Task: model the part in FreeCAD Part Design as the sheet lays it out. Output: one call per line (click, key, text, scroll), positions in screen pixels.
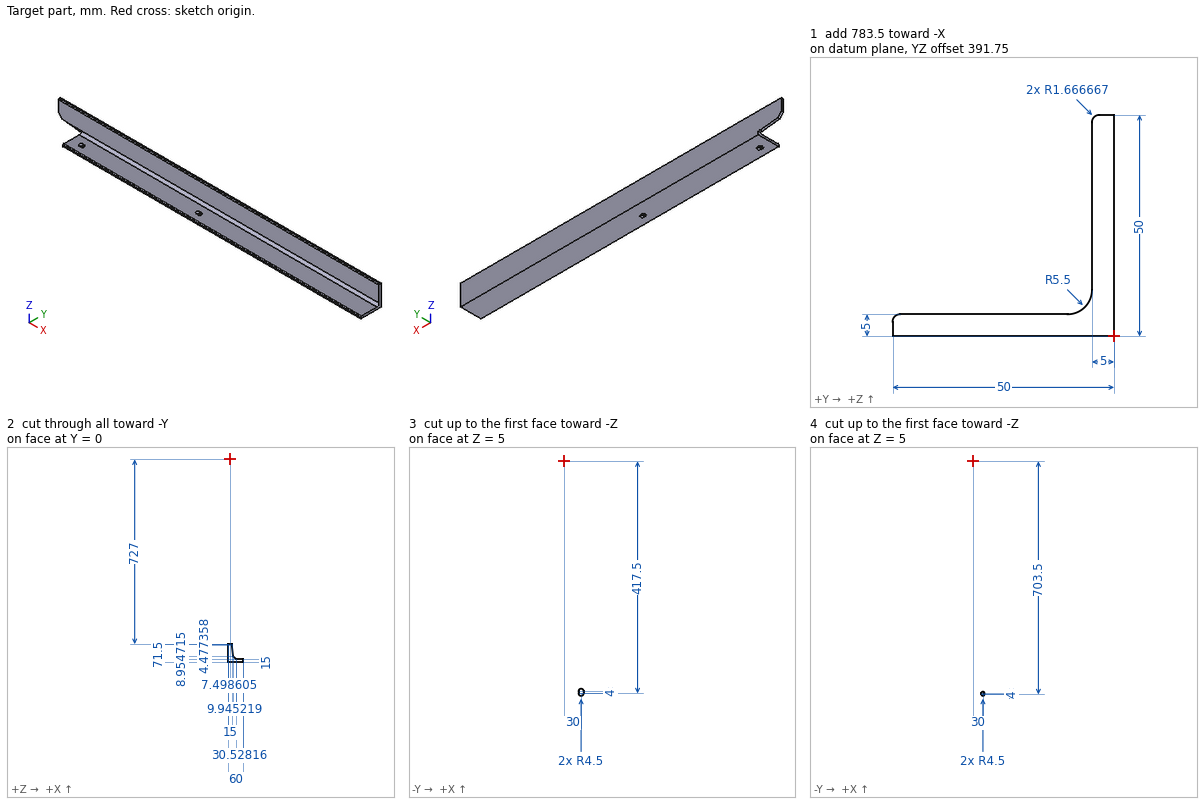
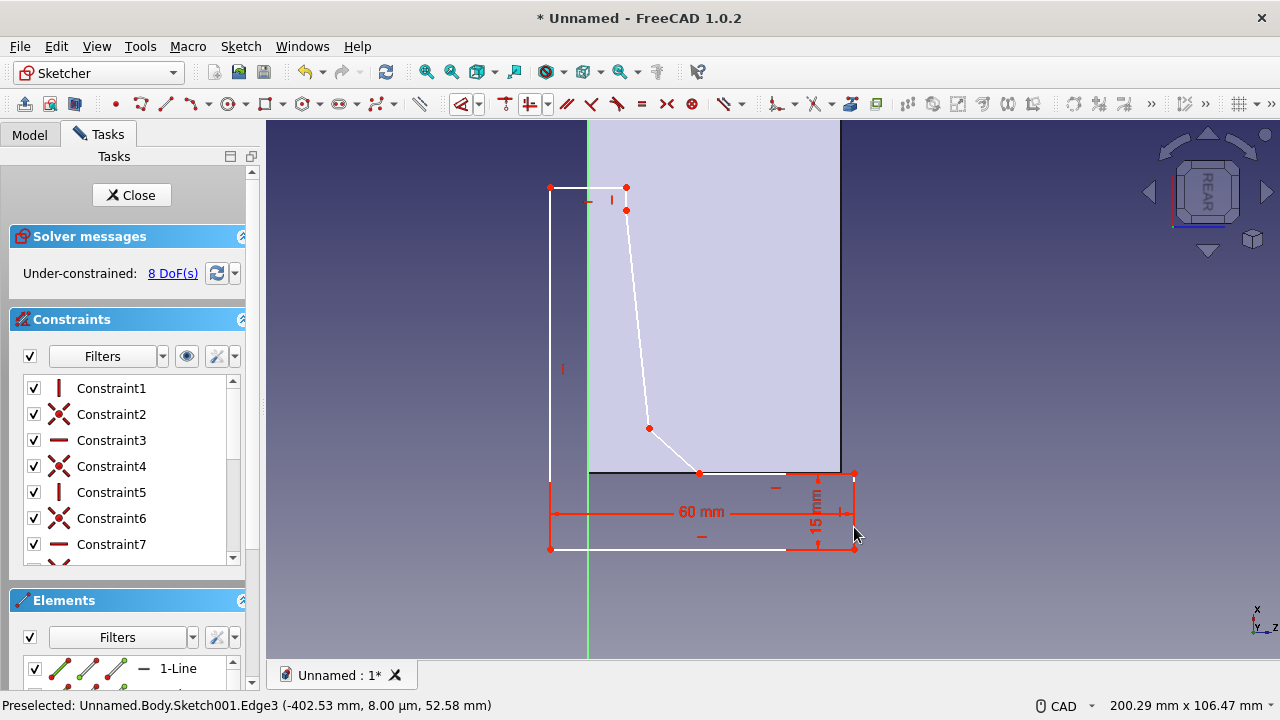
click(603, 188)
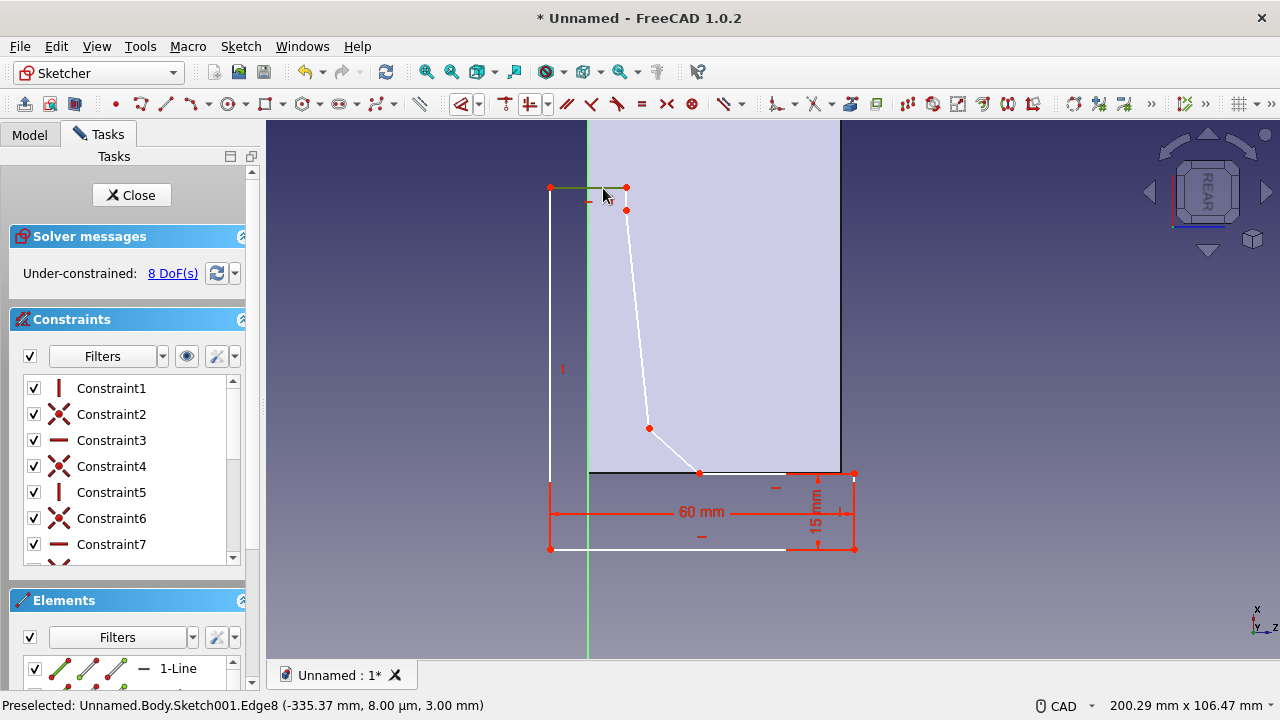
key(l)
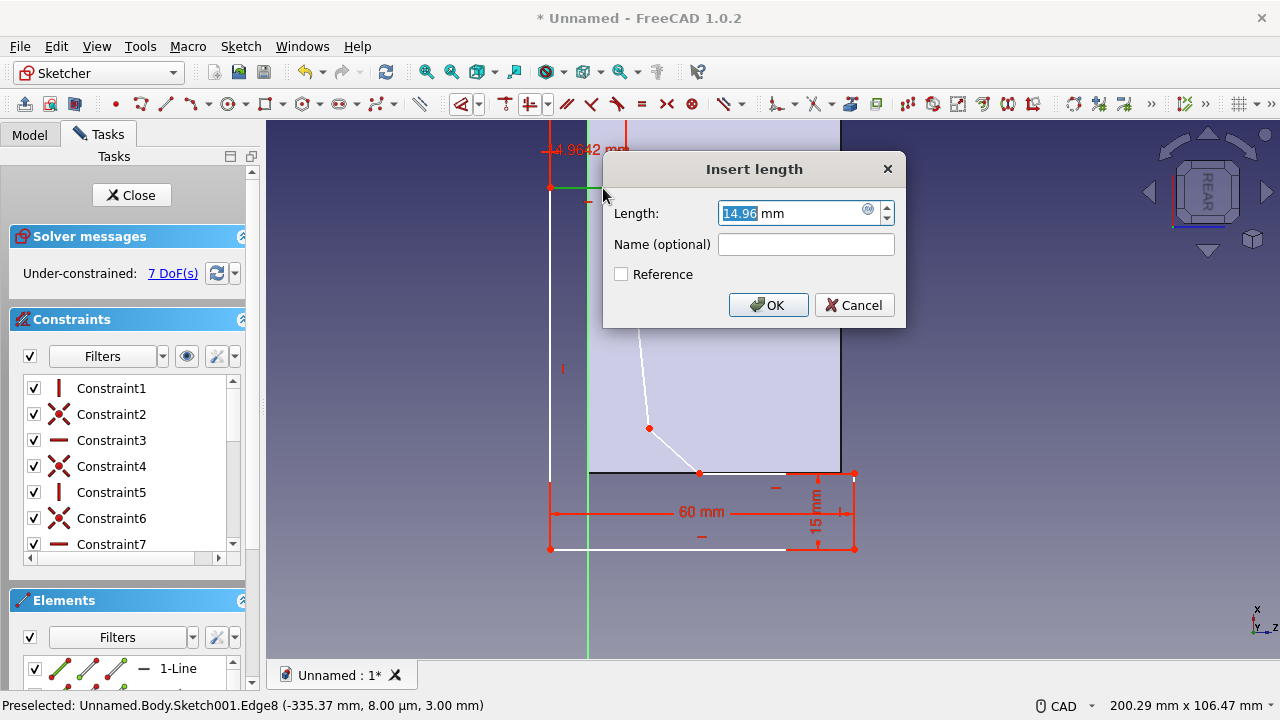
text(15)
key(Return)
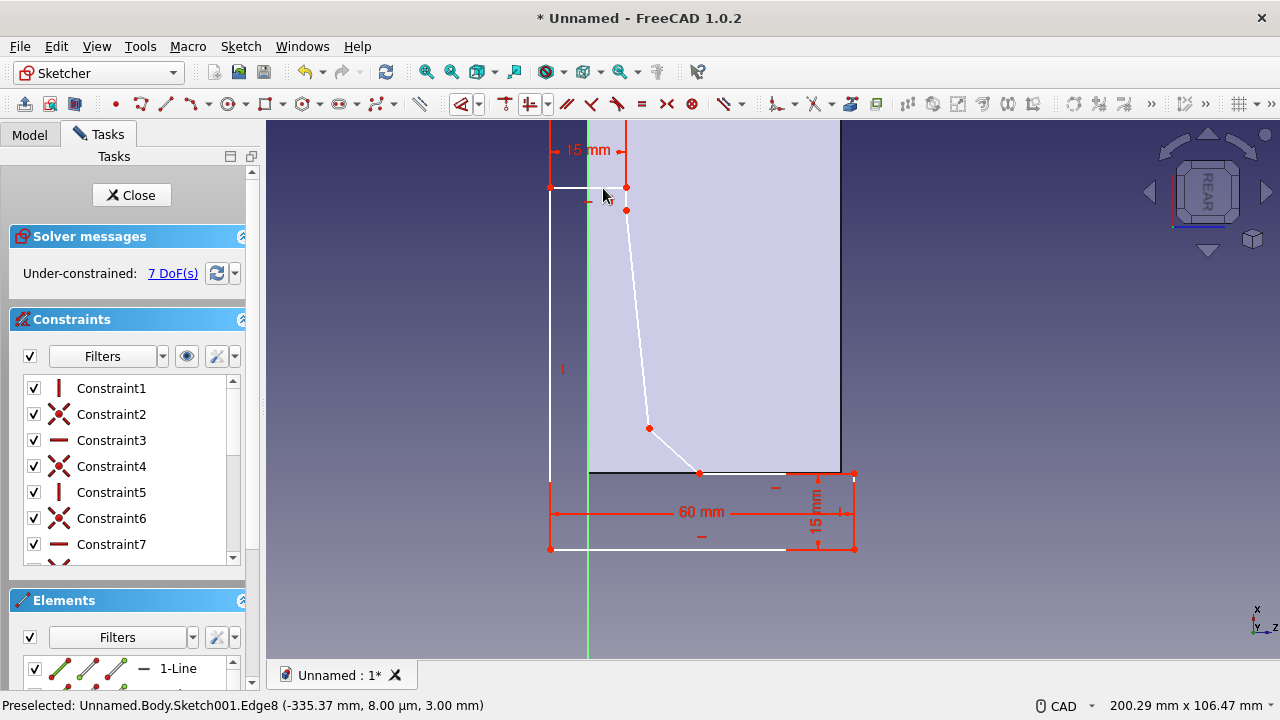
click(550, 297)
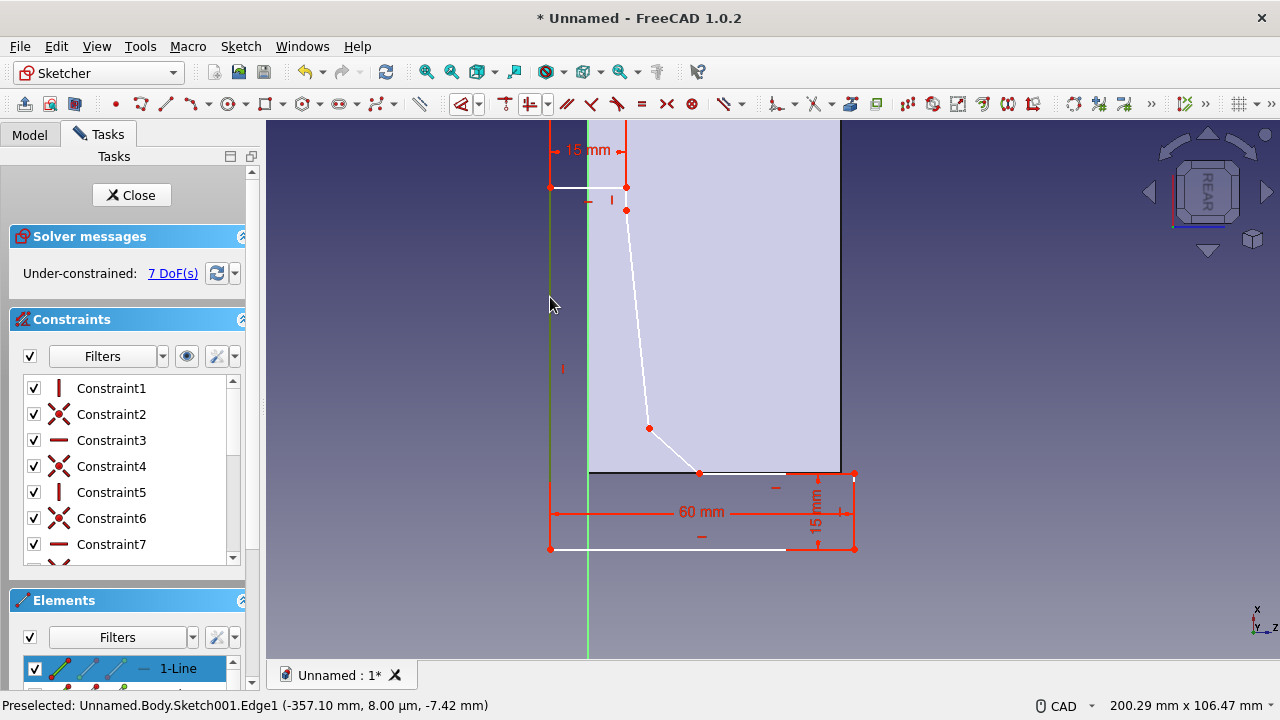
click(478, 104)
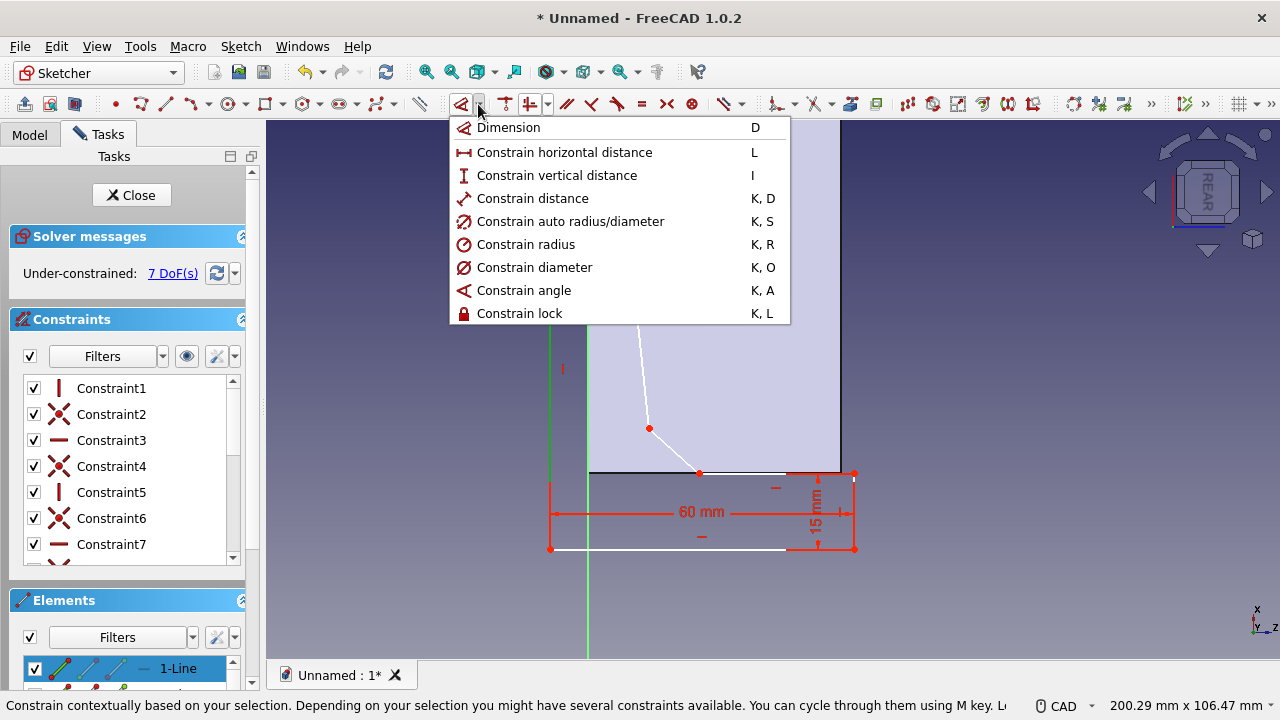
click(620, 176)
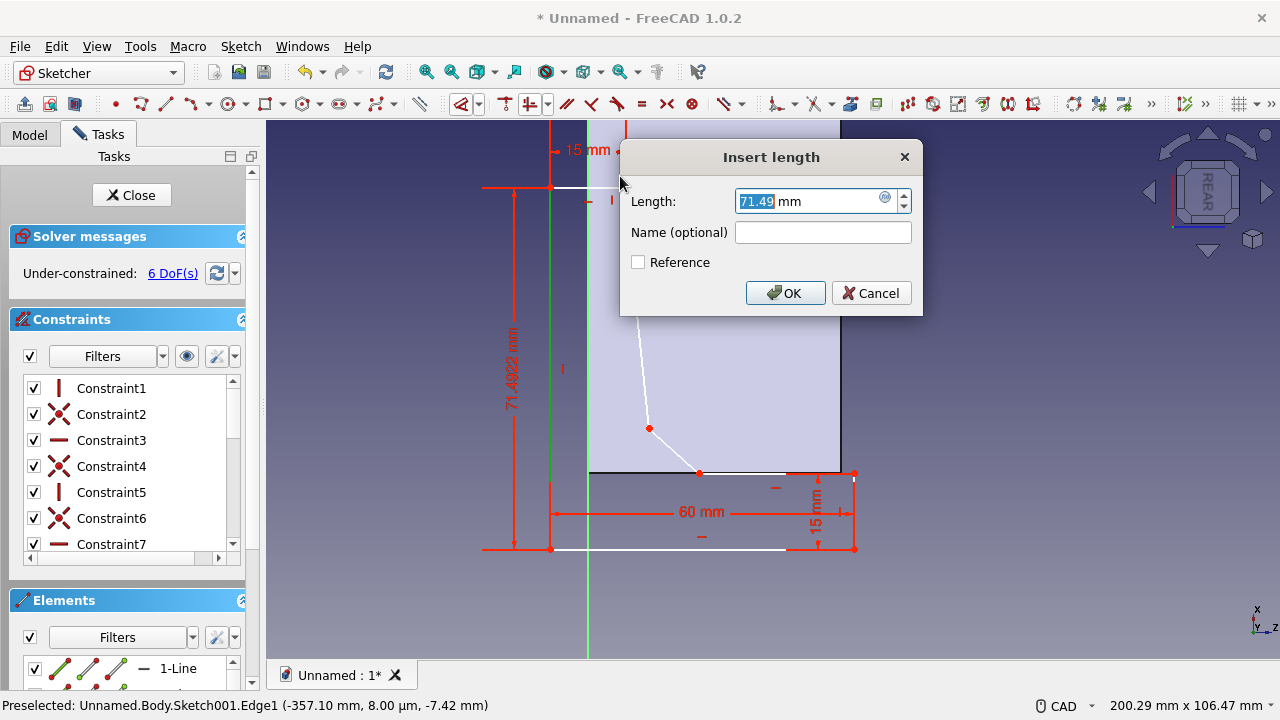
text(71.5)
key(Return)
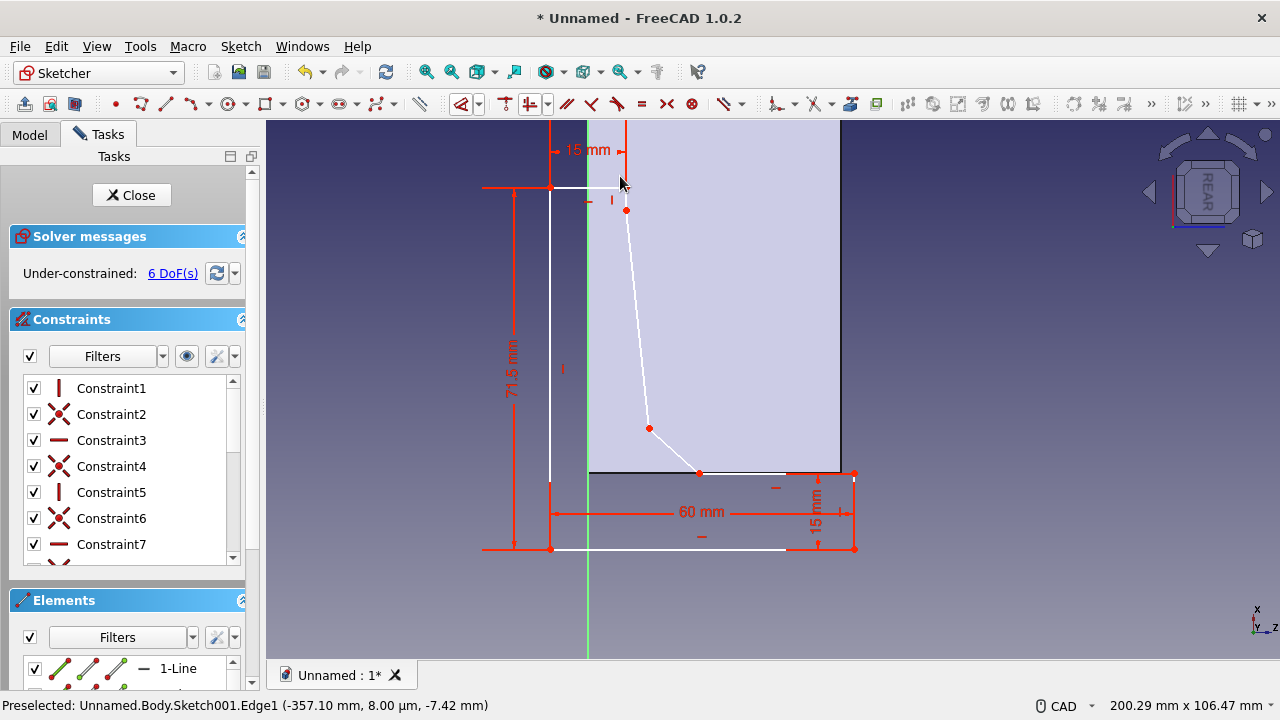
click(550, 188)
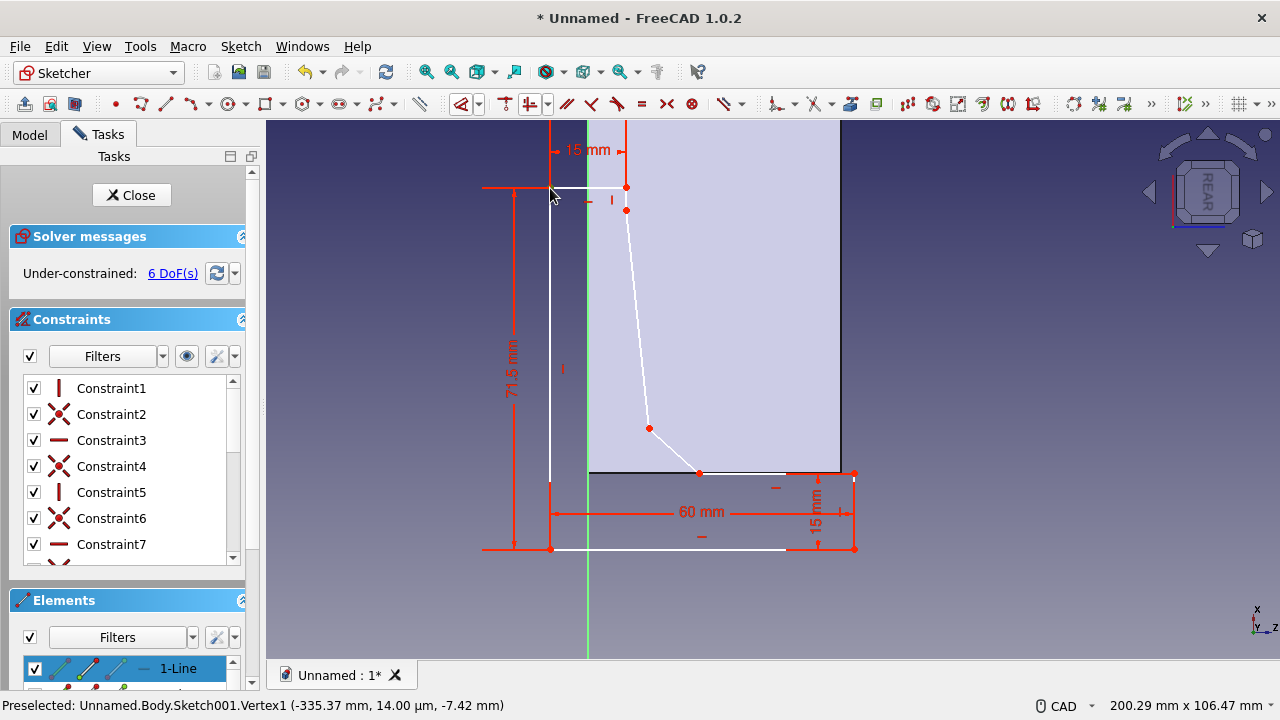
key(i)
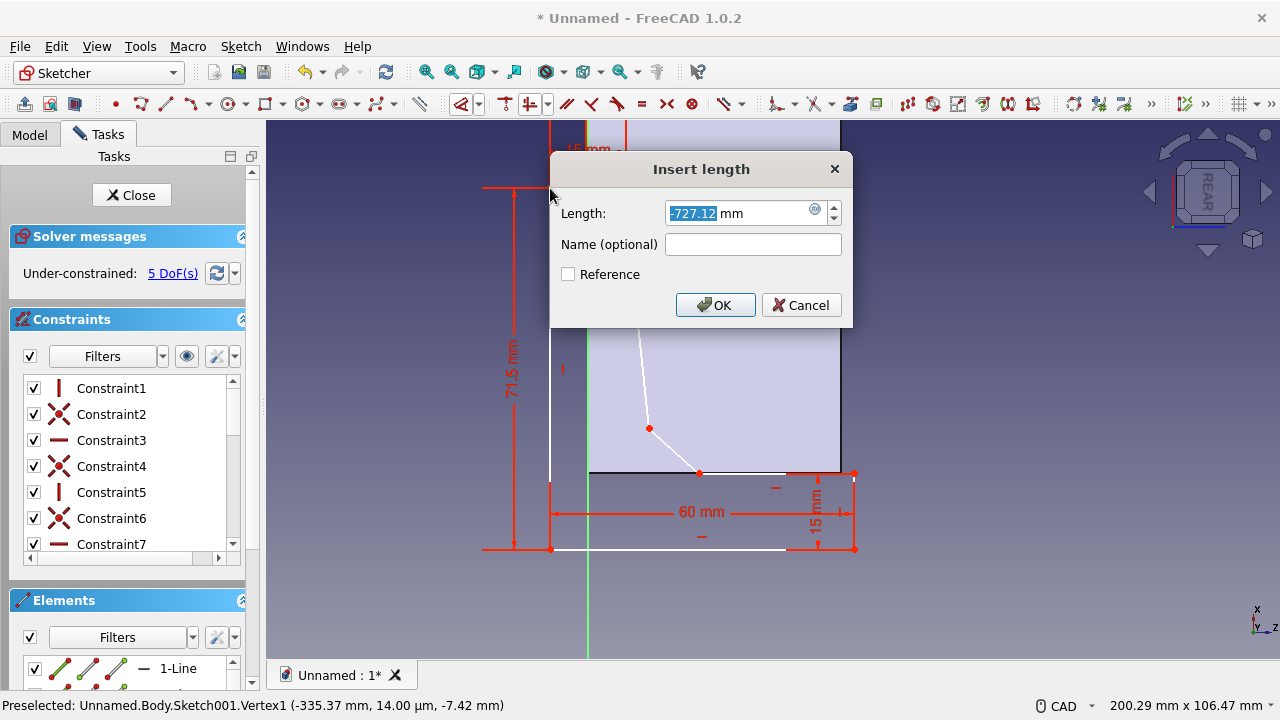
text(-727)
key(Return)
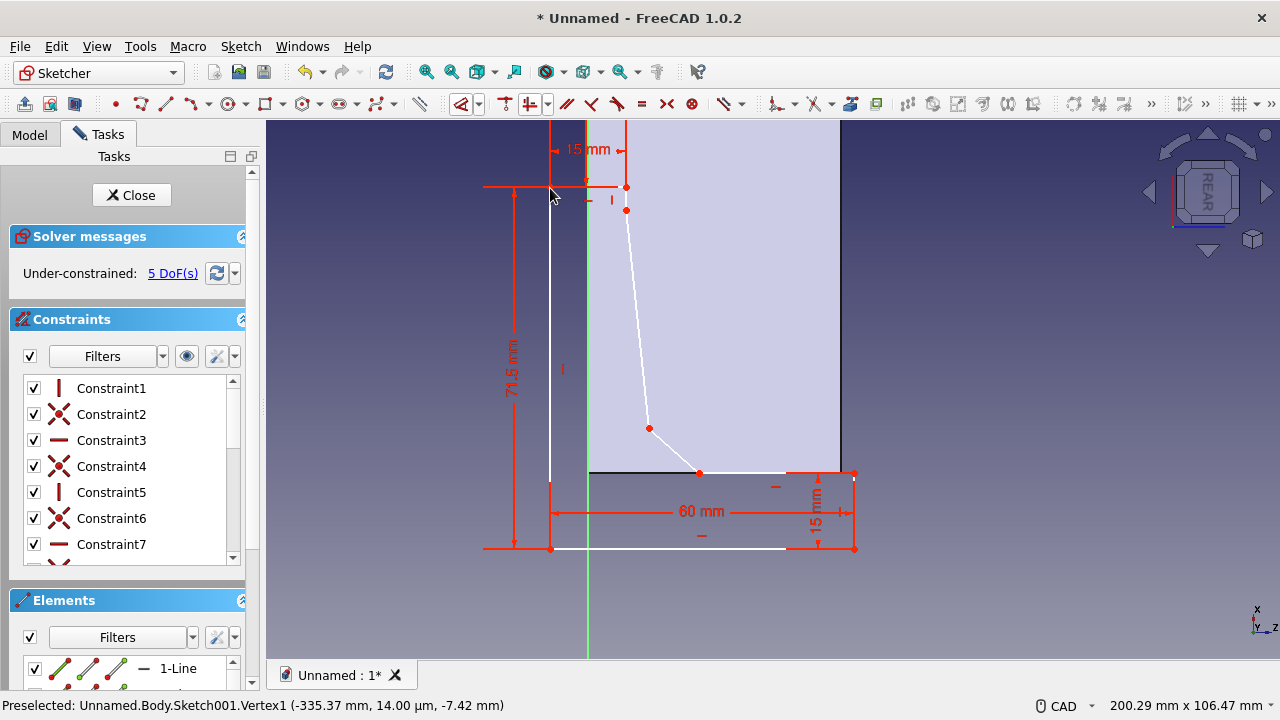
click(808, 473)